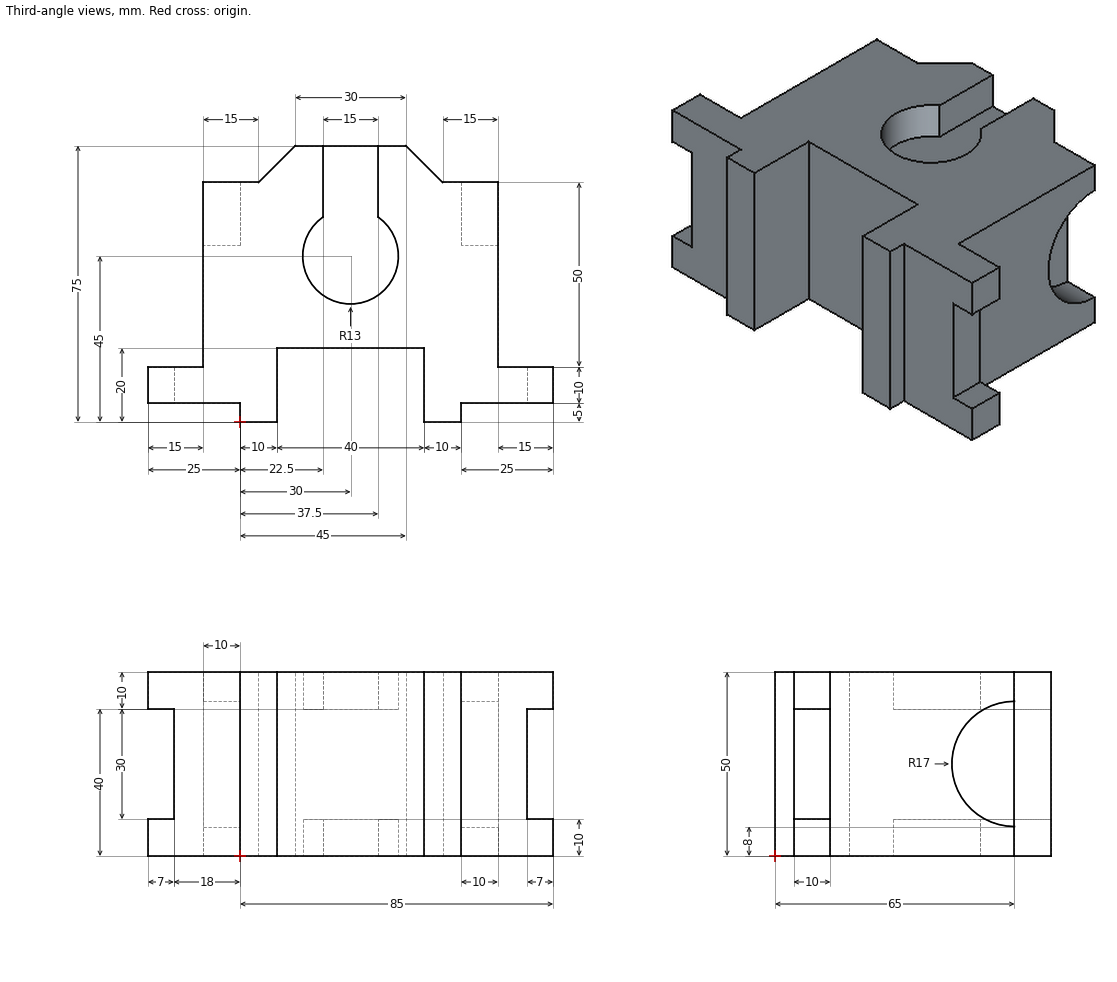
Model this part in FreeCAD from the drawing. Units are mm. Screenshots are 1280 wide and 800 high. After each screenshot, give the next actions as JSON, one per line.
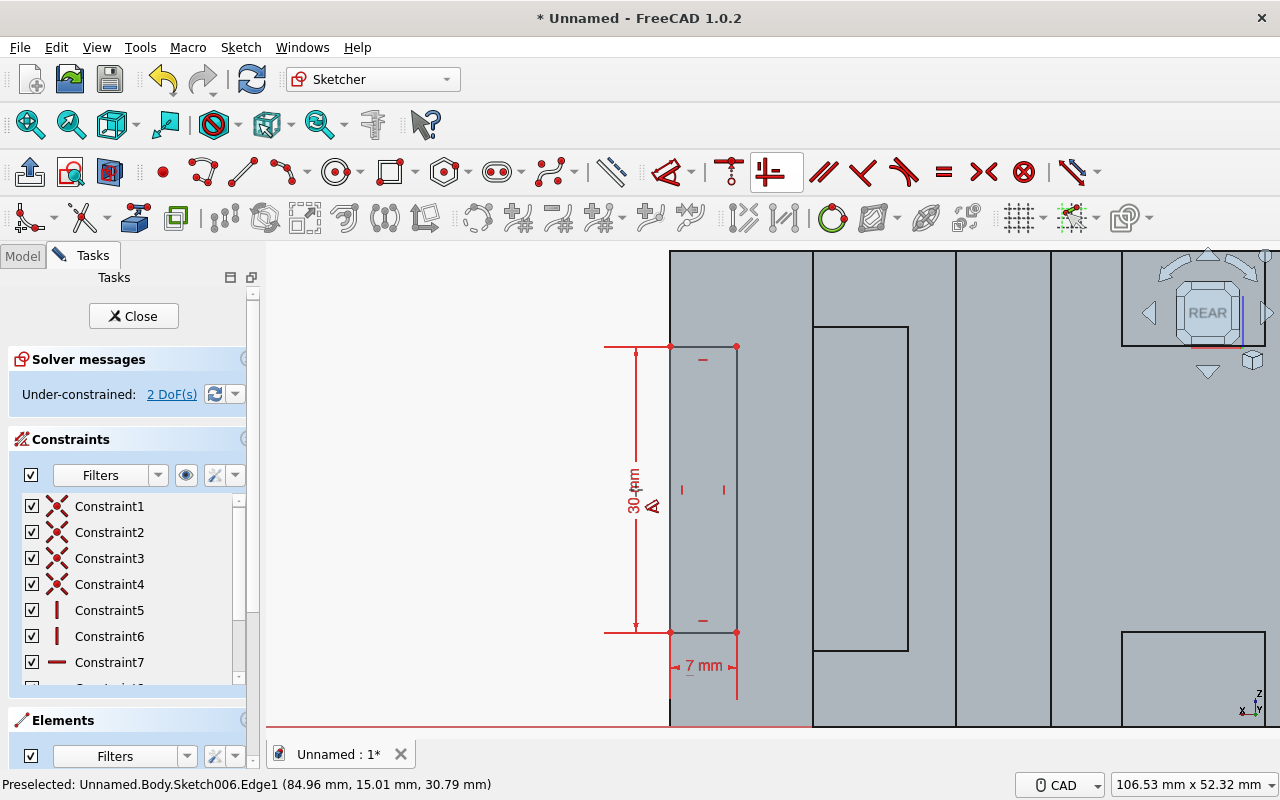
{"action": "left_click", "coordinate": [670, 347]}
{"action": "left_click", "coordinate": [893, 313]}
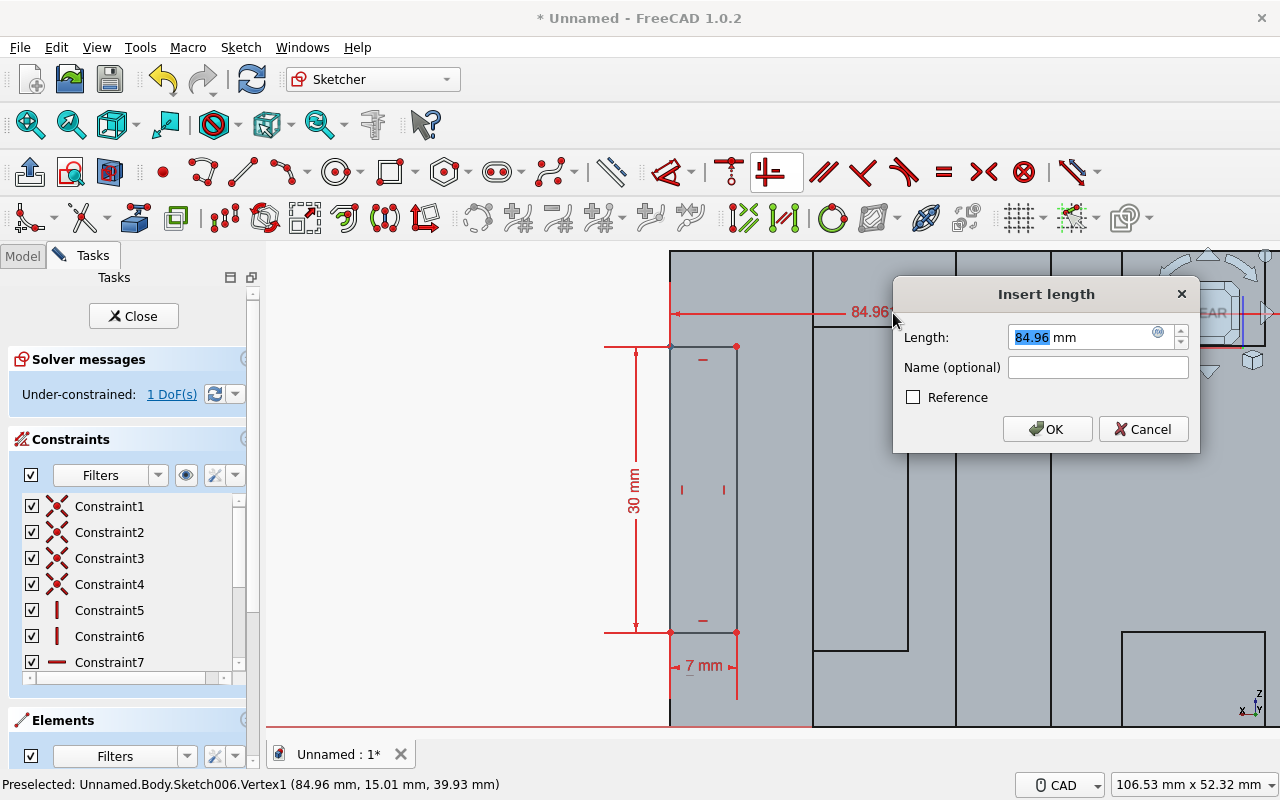
{"action": "type", "text": "85"}
{"action": "key", "text": "Return"}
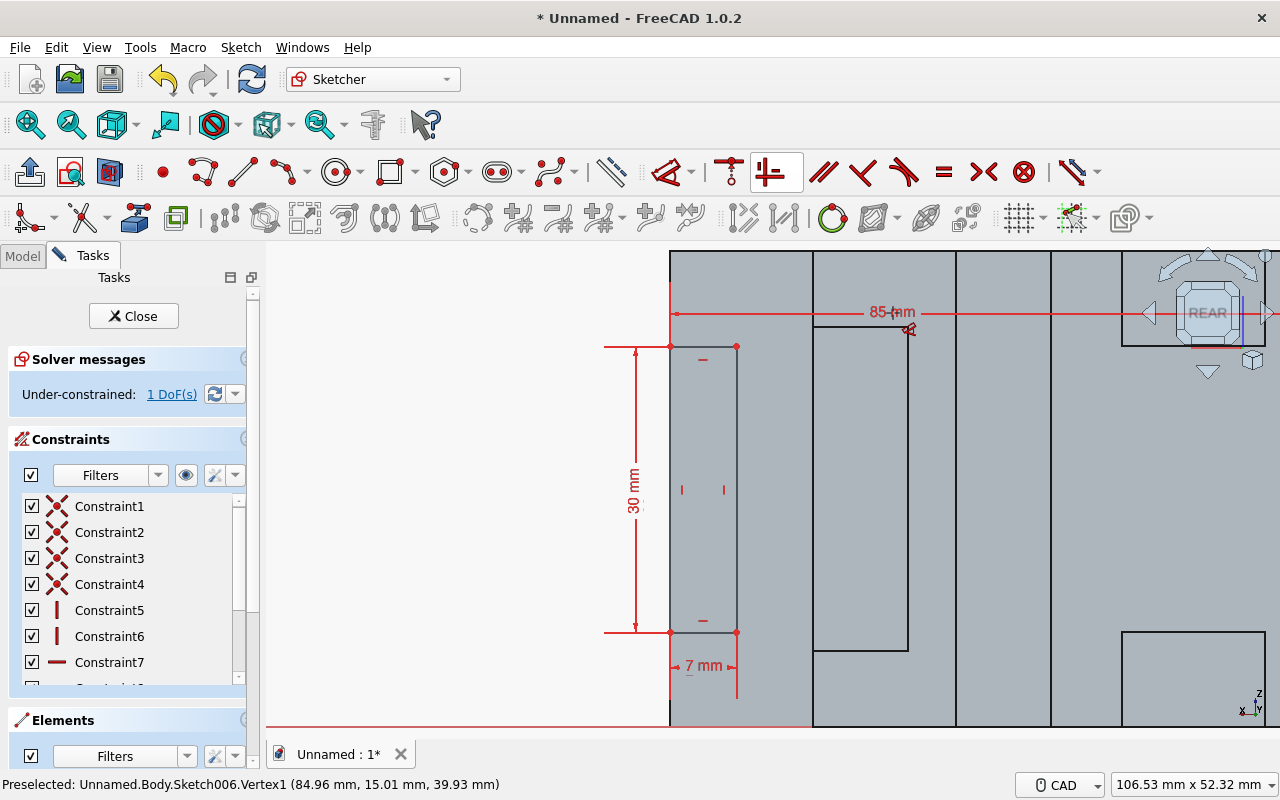
{"action": "left_click", "coordinate": [670, 347]}
{"action": "left_click", "coordinate": [636, 529]}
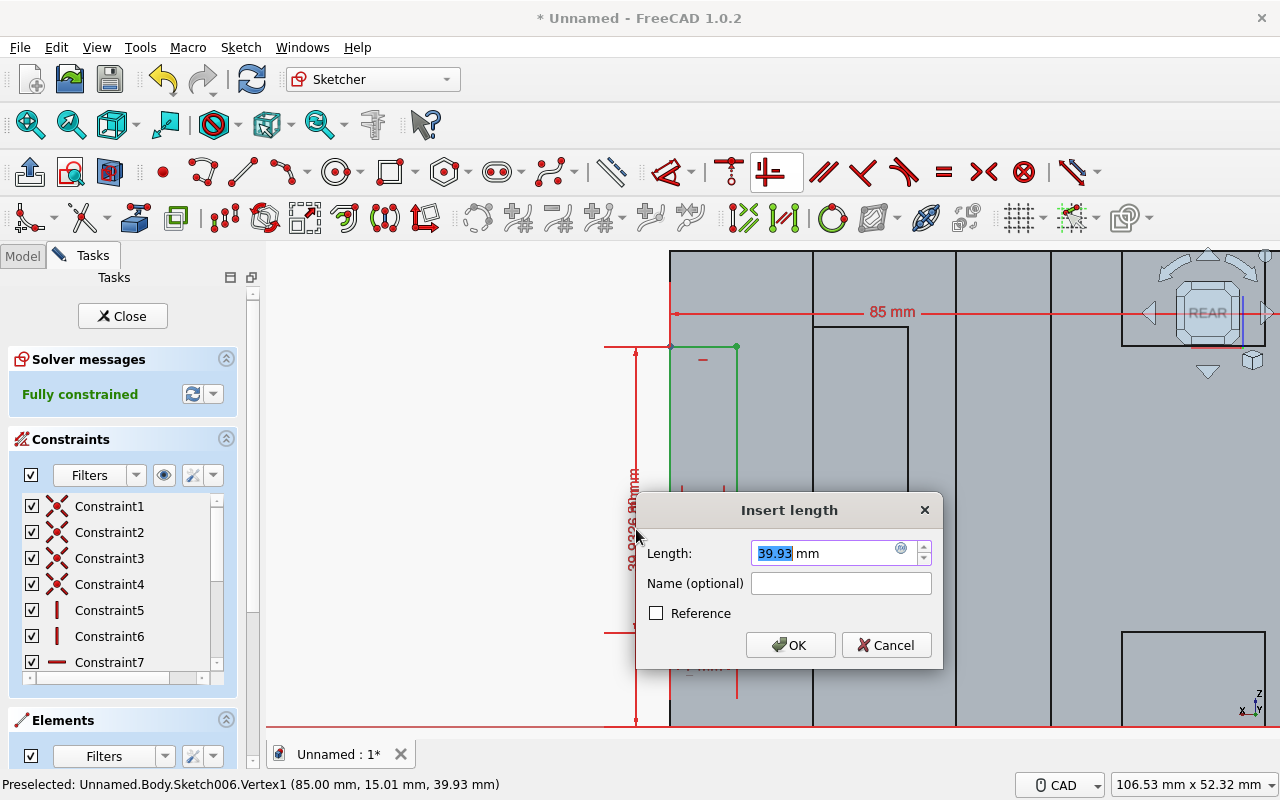
{"action": "type", "text": "40"}
{"action": "key", "text": "Return"}
{"action": "key", "text": "Escape"}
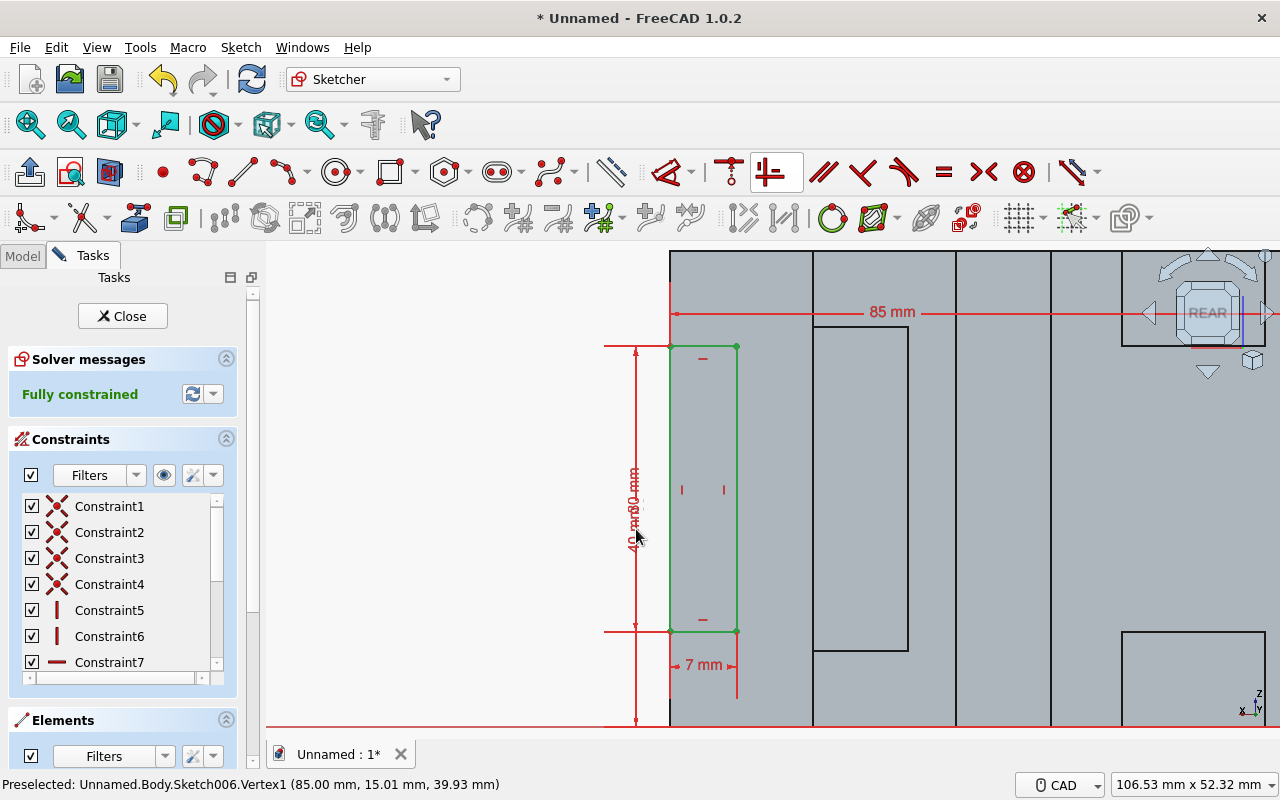
{"action": "left_click", "coordinate": [123, 316]}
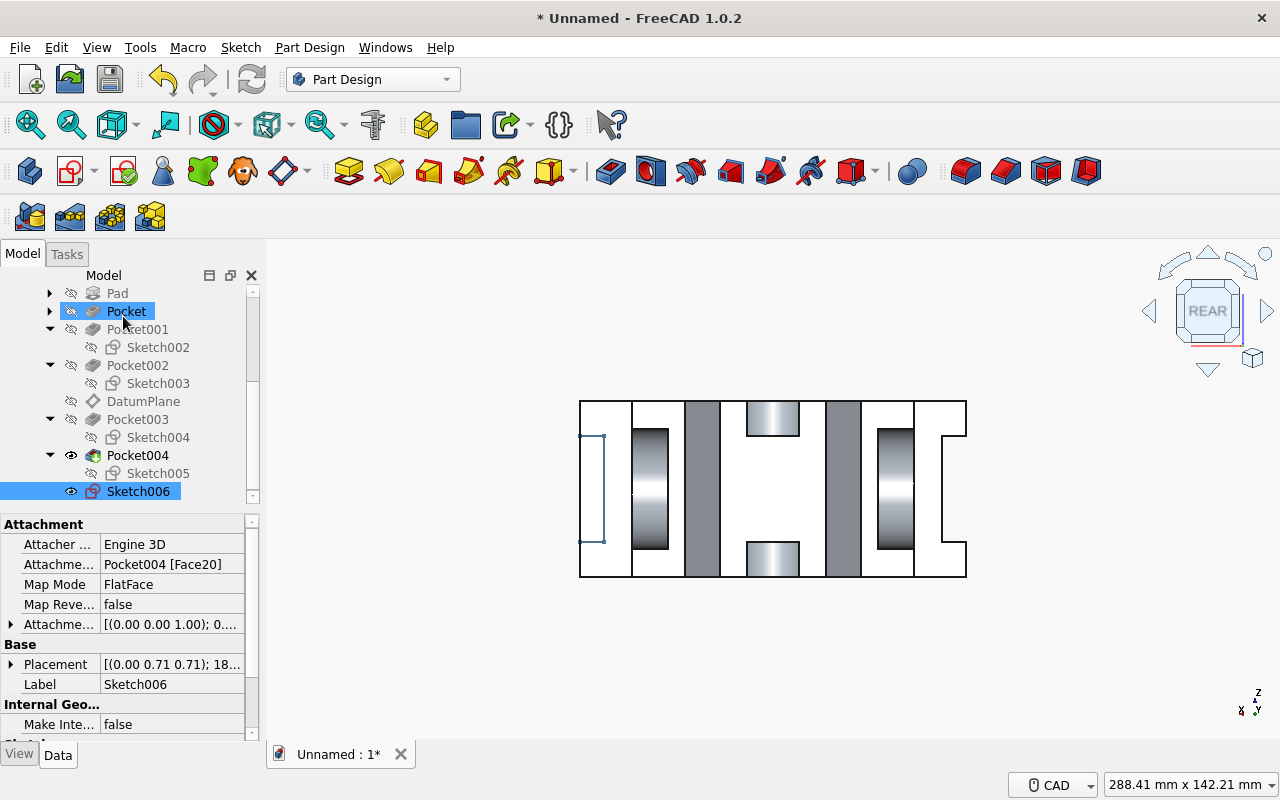
{"action": "left_click", "coordinate": [612, 172]}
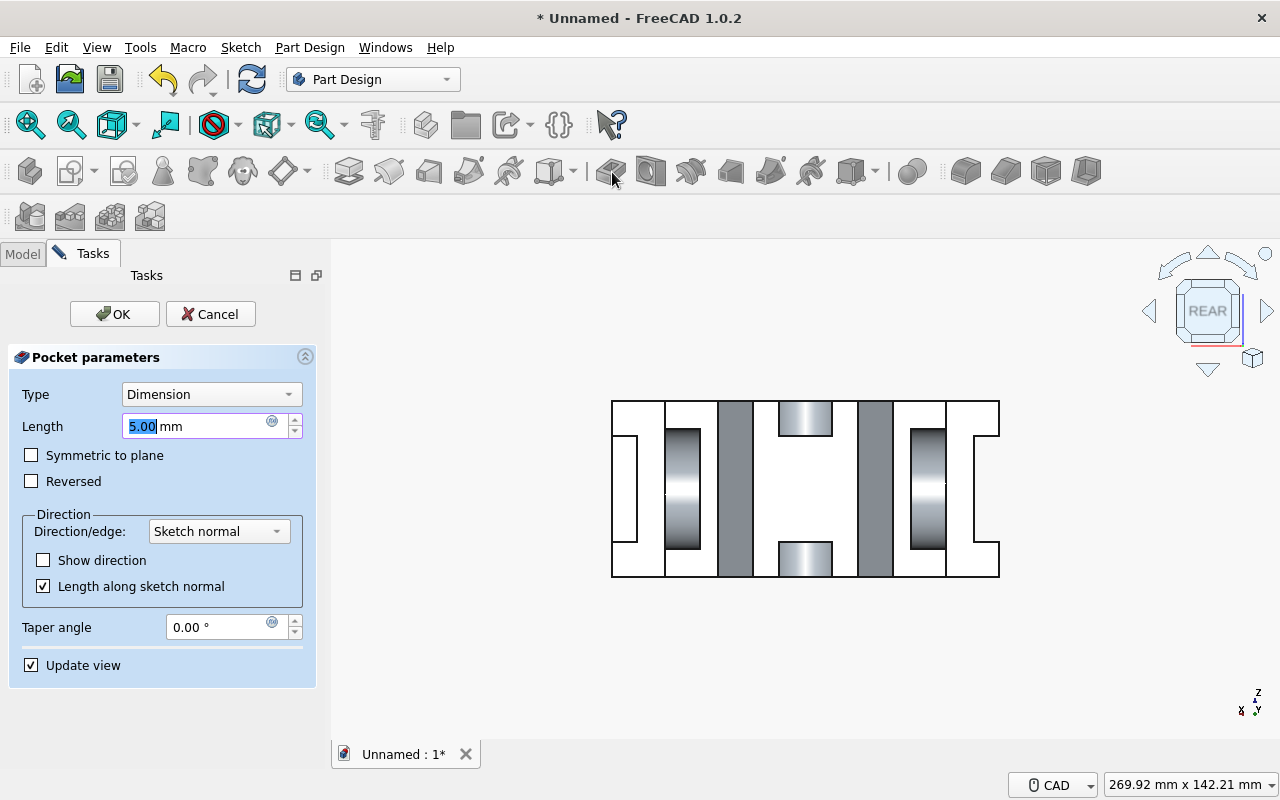
{"action": "type", "text": "10"}
{"action": "key", "text": "Tab"}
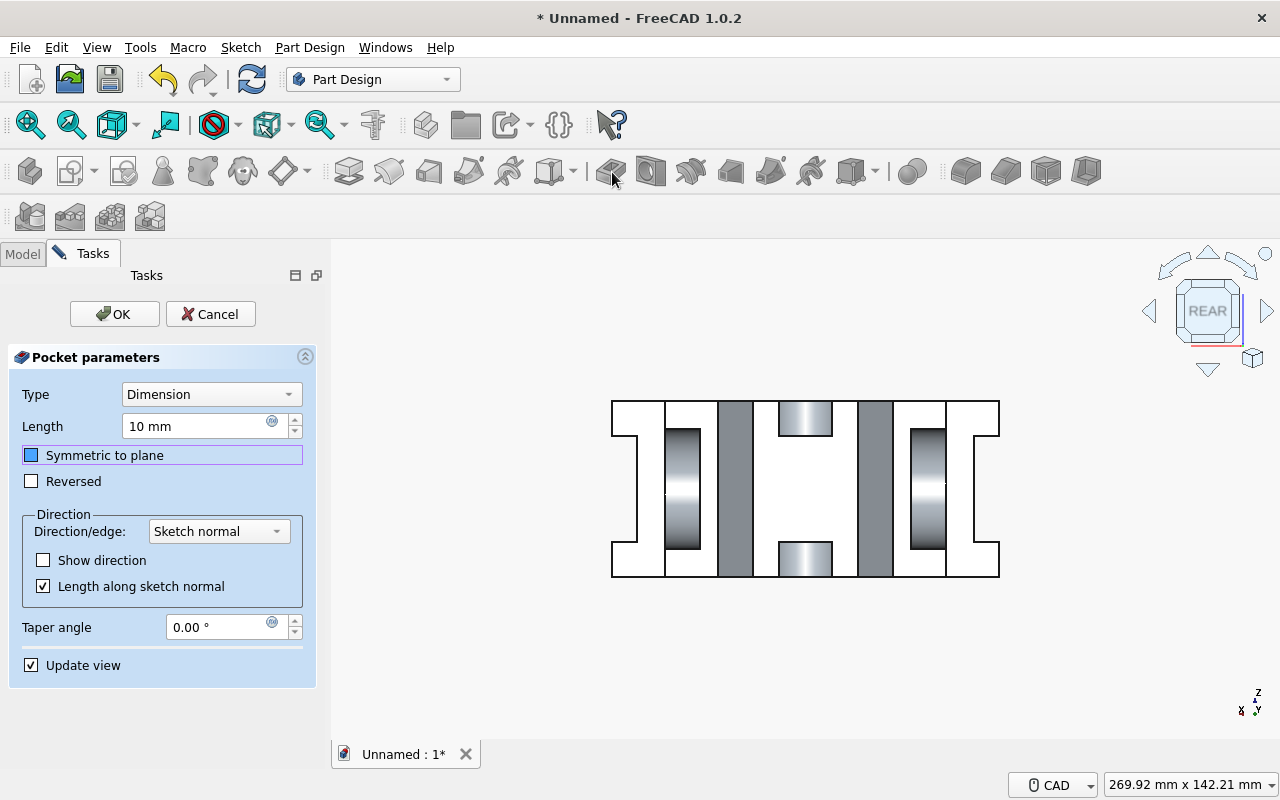
{"action": "left_click", "coordinate": [115, 314]}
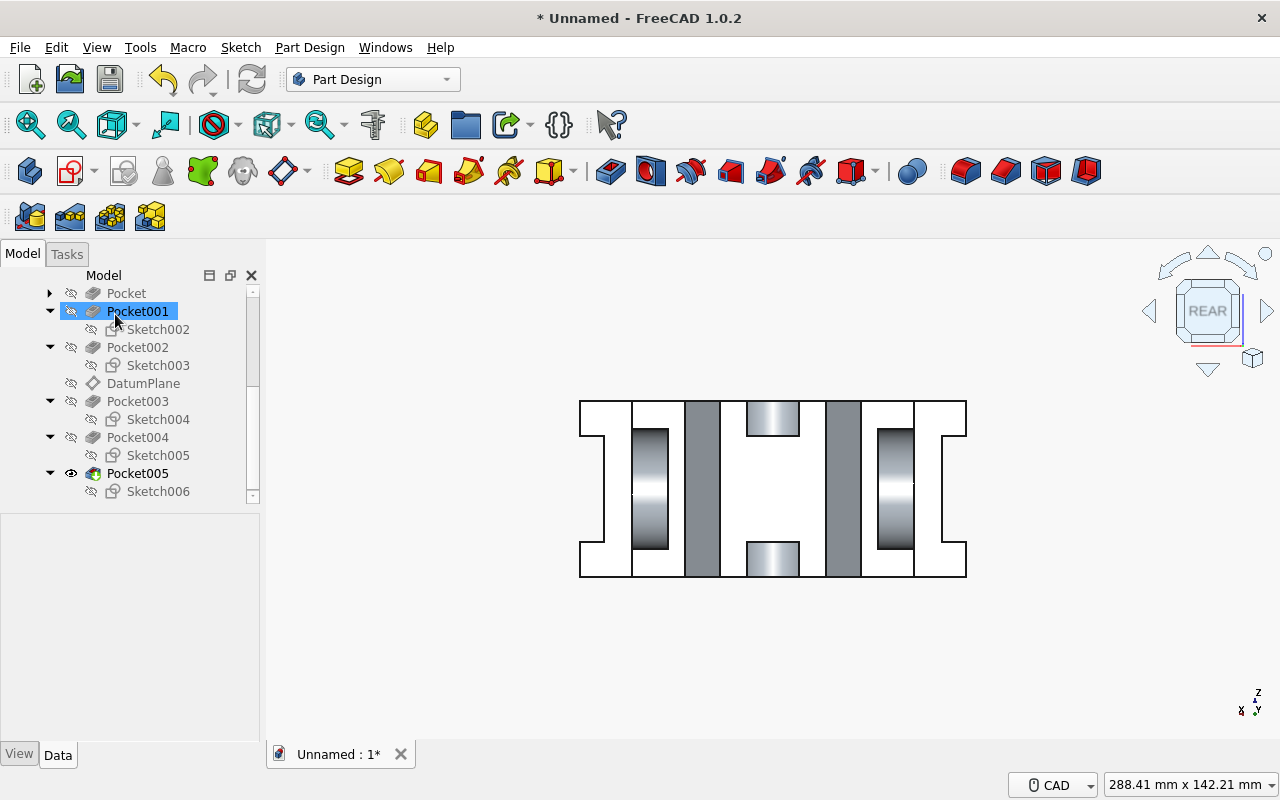
{"action": "key", "text": "0"}